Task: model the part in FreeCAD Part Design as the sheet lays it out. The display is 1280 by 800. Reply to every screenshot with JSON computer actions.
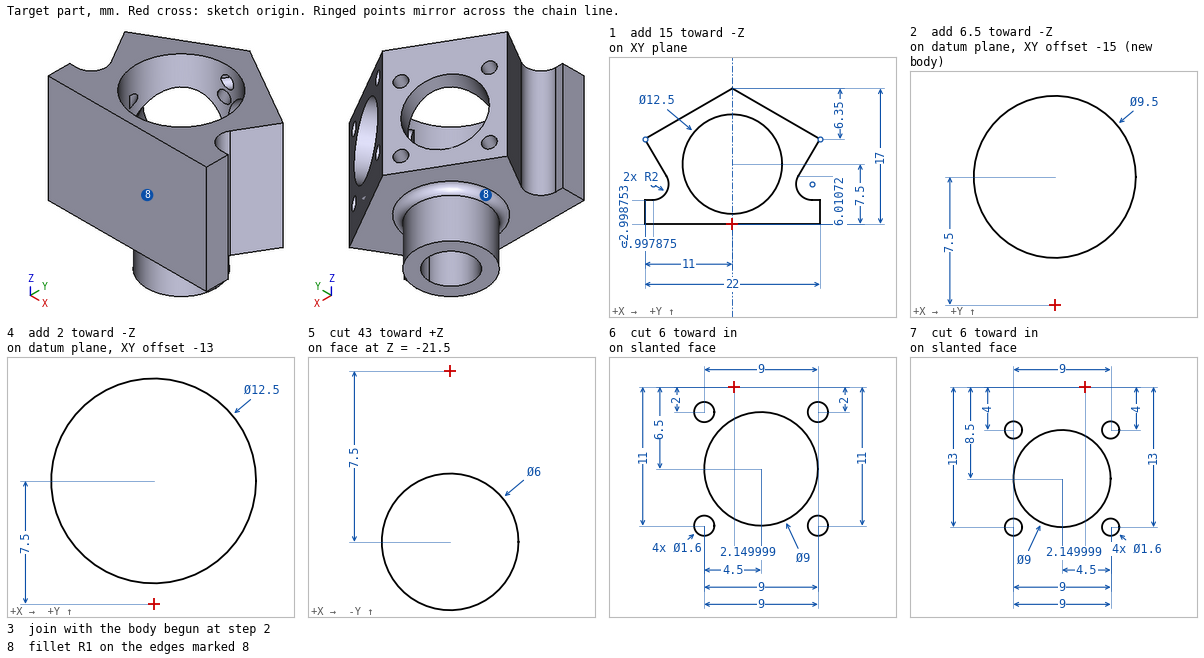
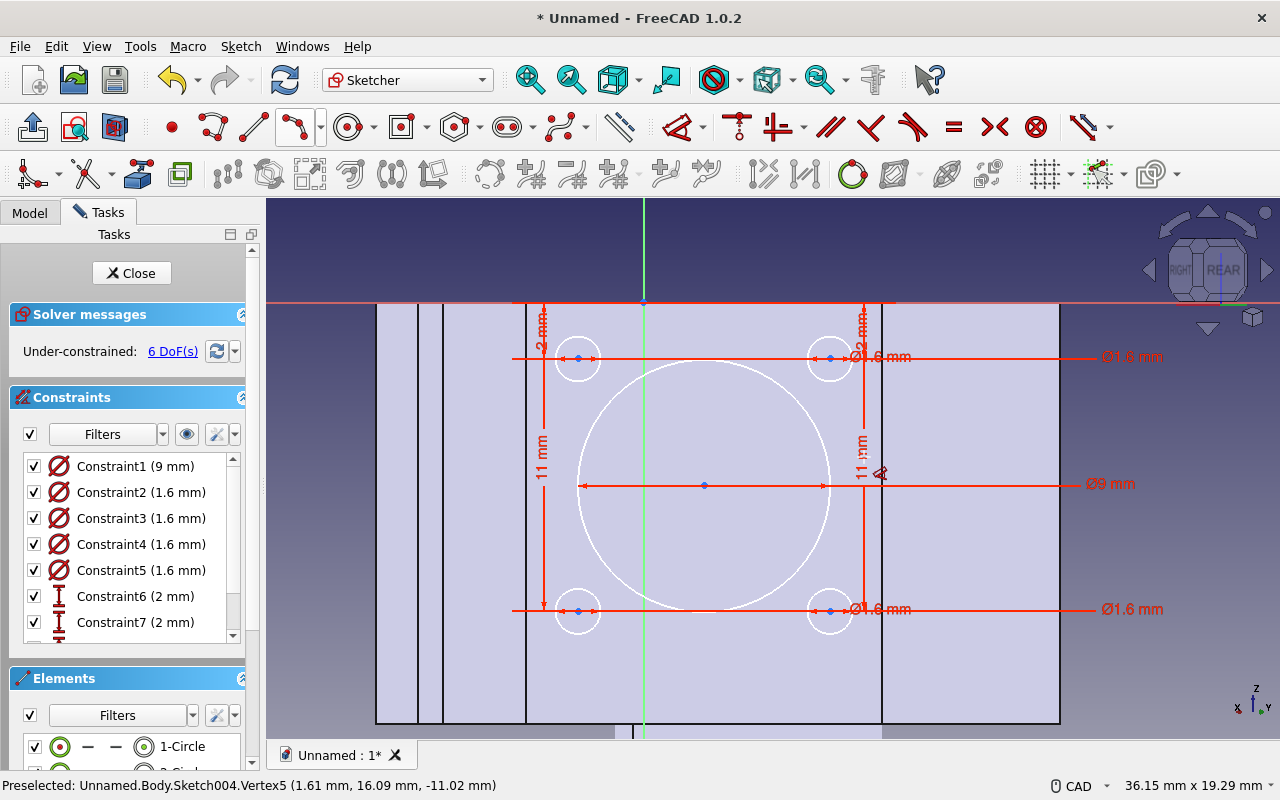
{"action": "left_click", "coordinate": [578, 359]}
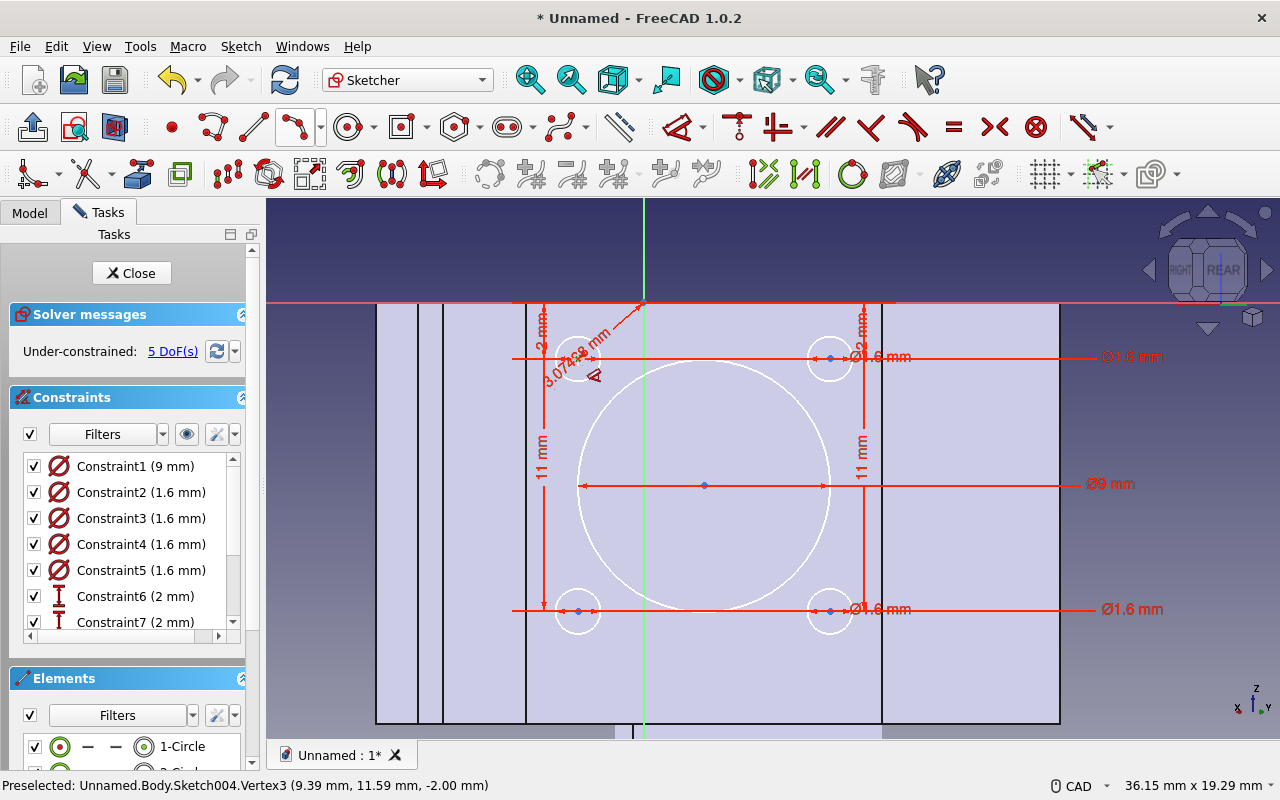
{"action": "left_click", "coordinate": [830, 359]}
{"action": "left_click", "coordinate": [704, 325]}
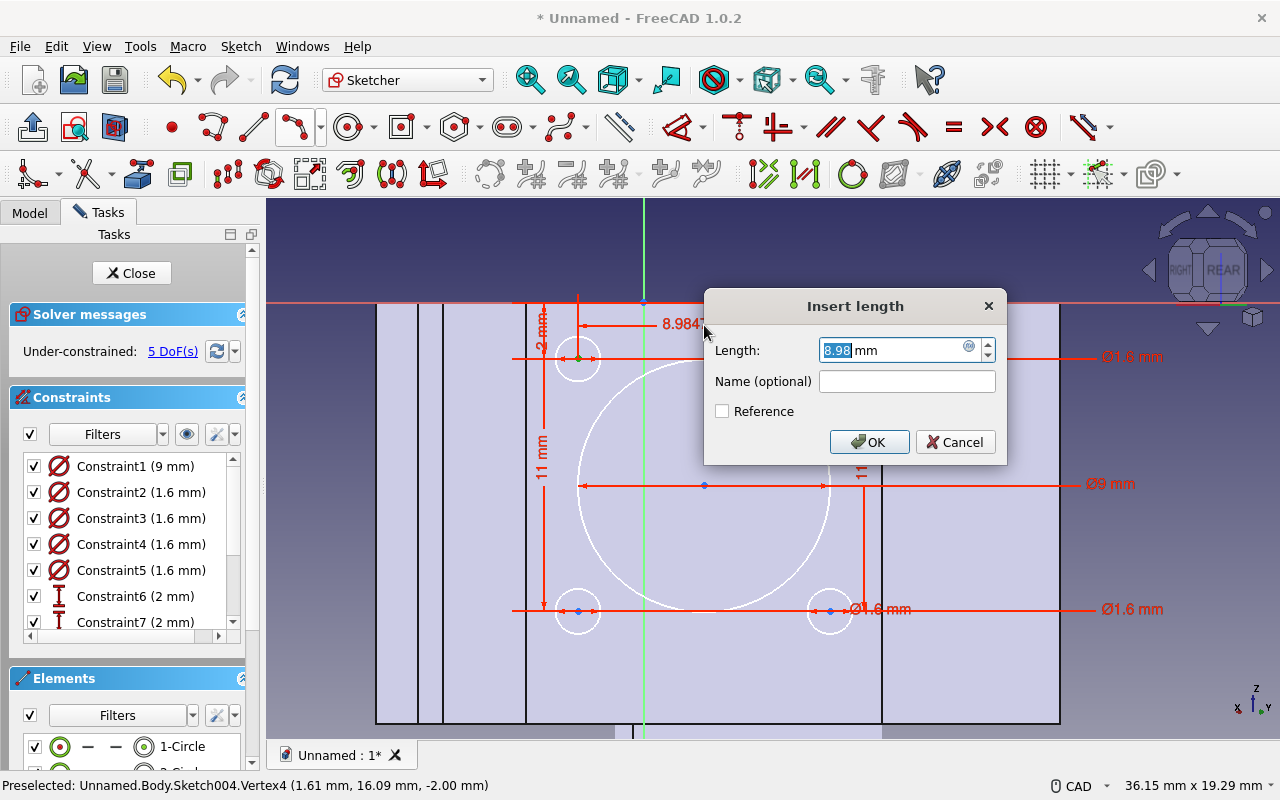
{"action": "type", "text": "9"}
{"action": "key", "text": "Return"}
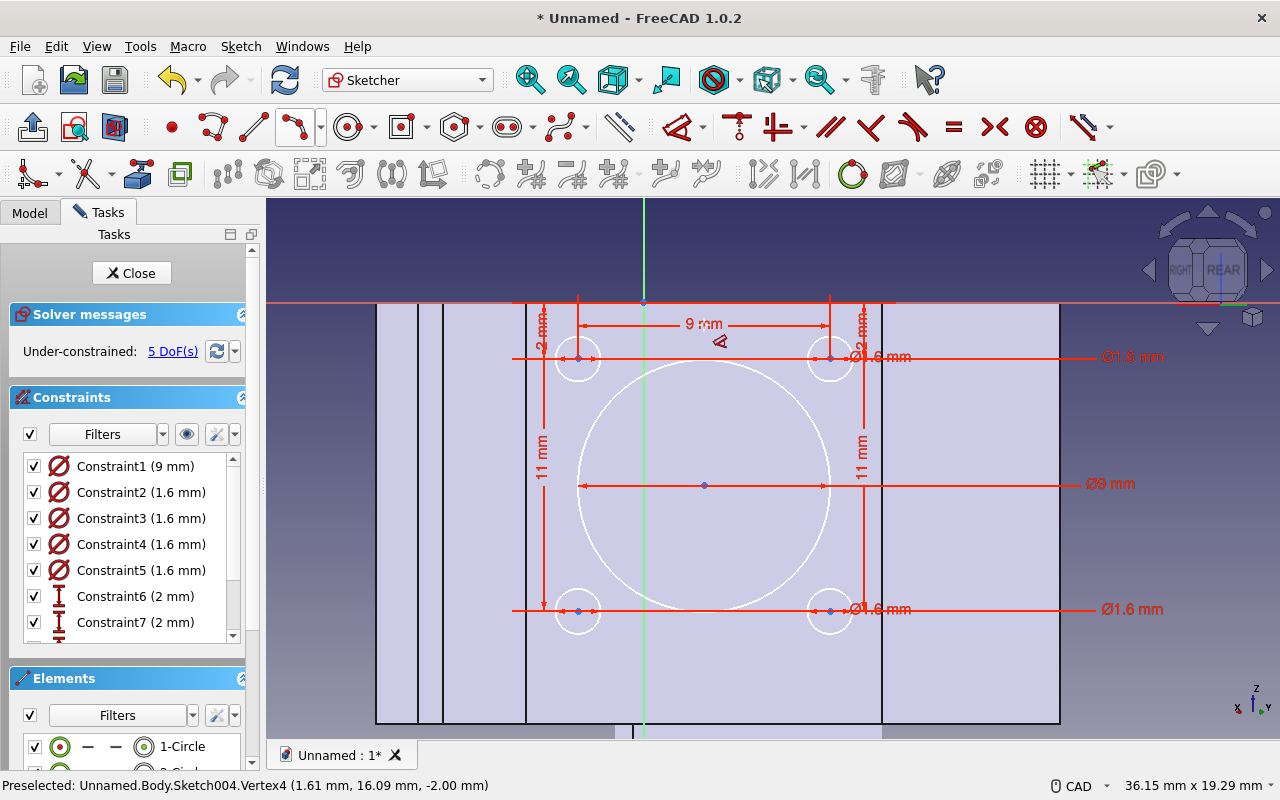
{"action": "left_click", "coordinate": [578, 611]}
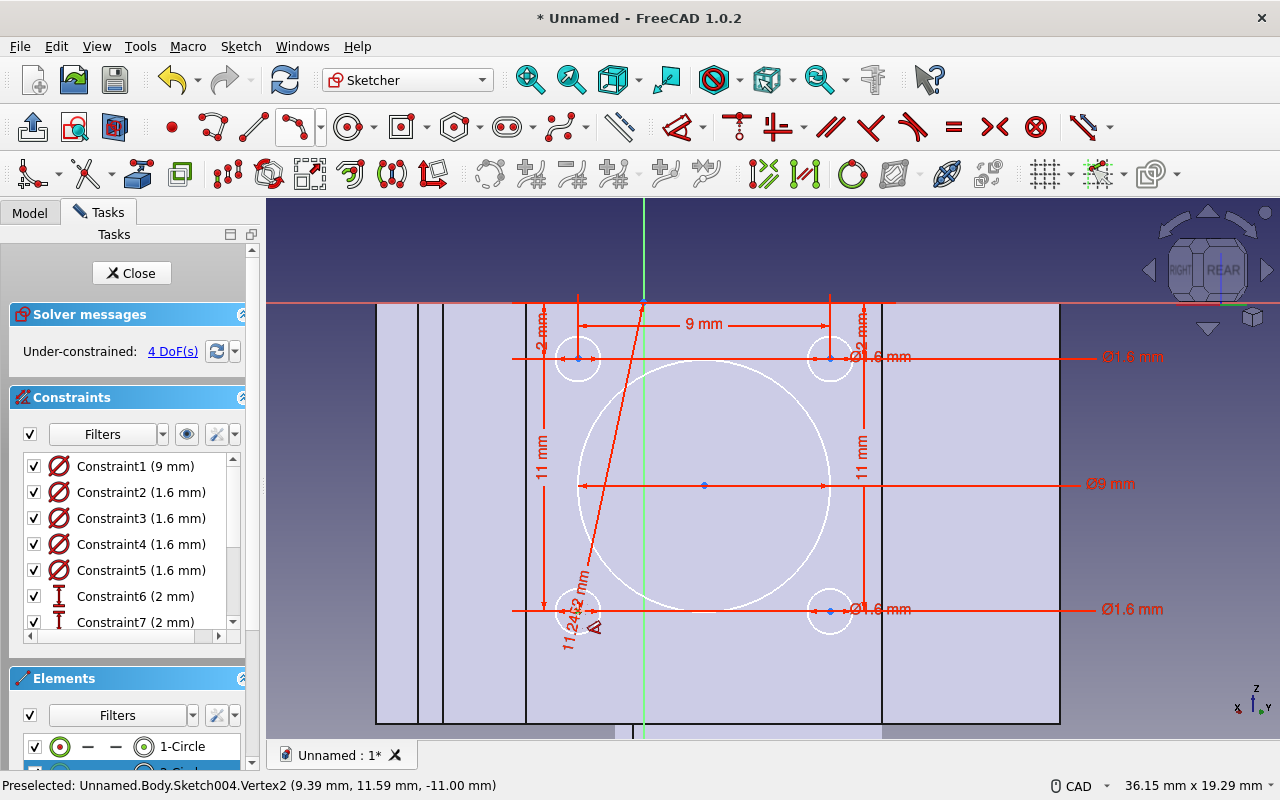
{"action": "left_click", "coordinate": [830, 359]}
{"action": "left_click", "coordinate": [704, 645]}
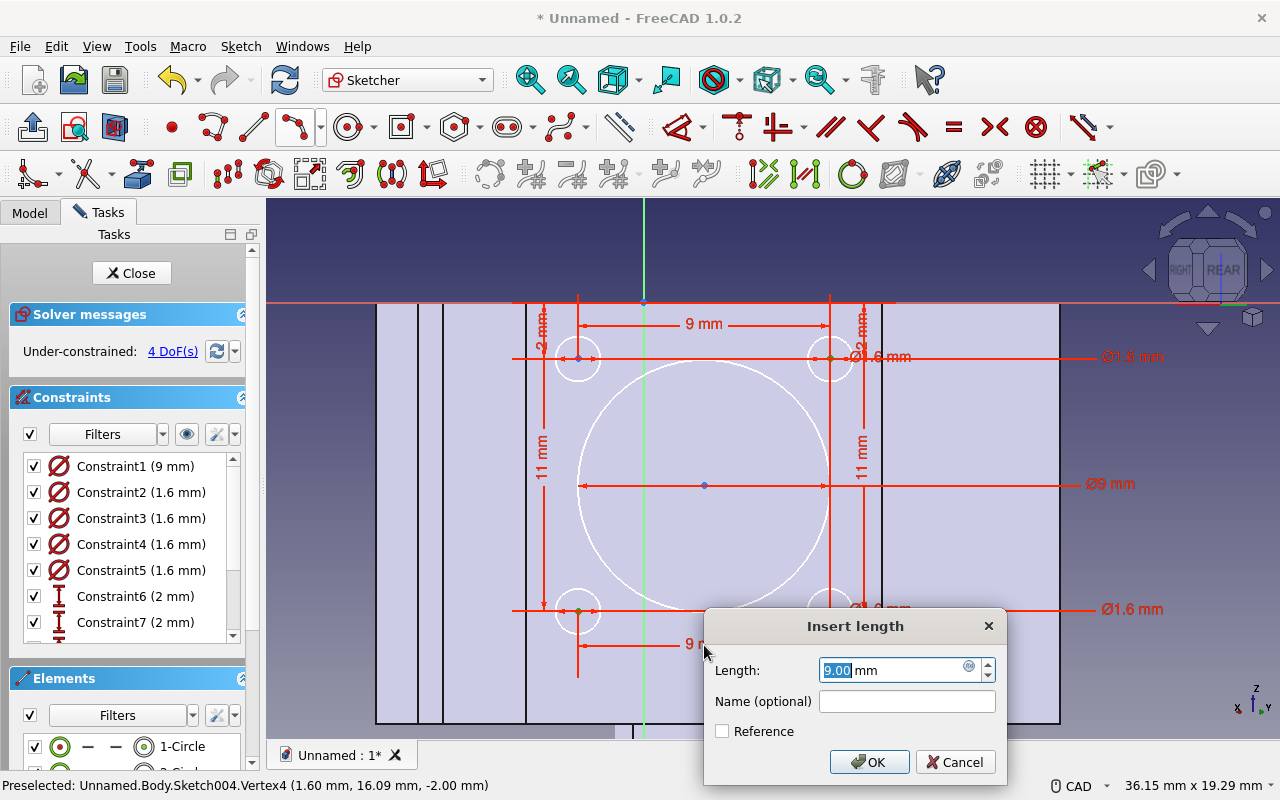
{"action": "type", "text": "9"}
{"action": "key", "text": "Return"}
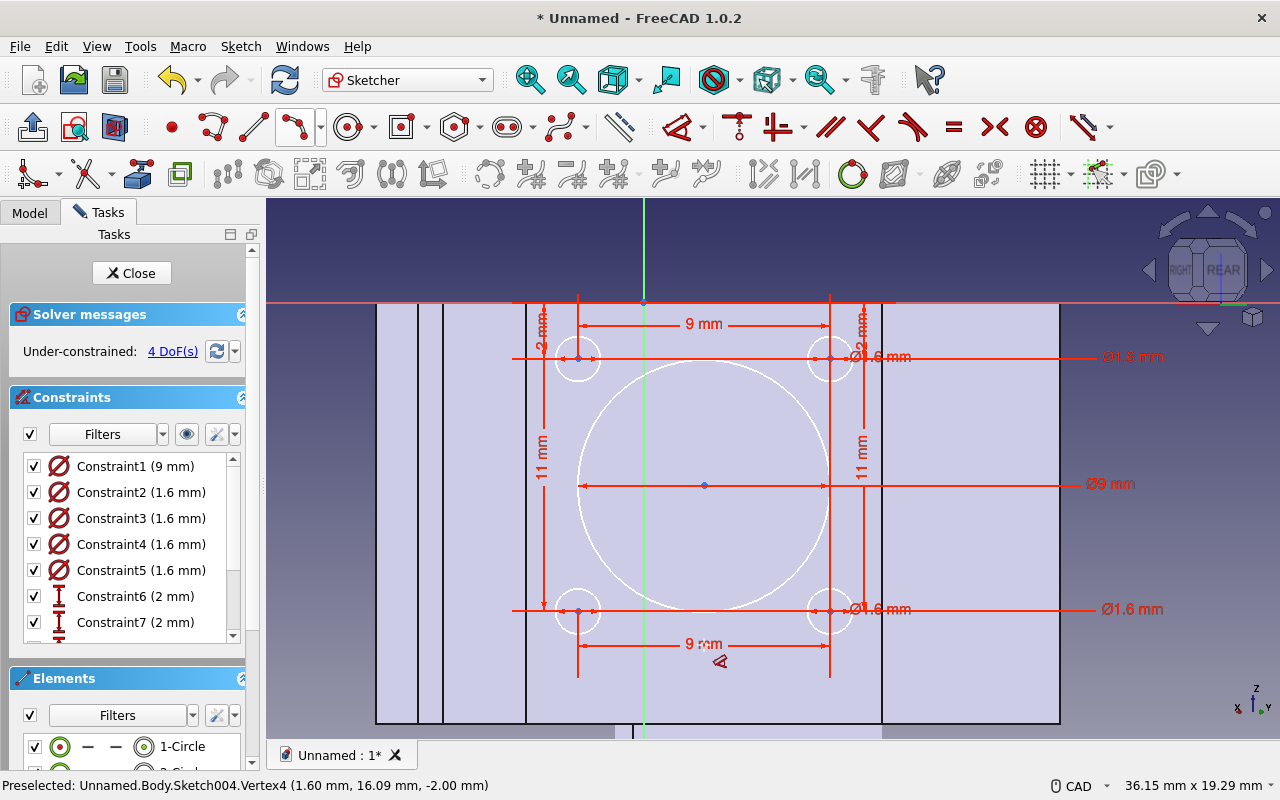
{"action": "left_click", "coordinate": [578, 611]}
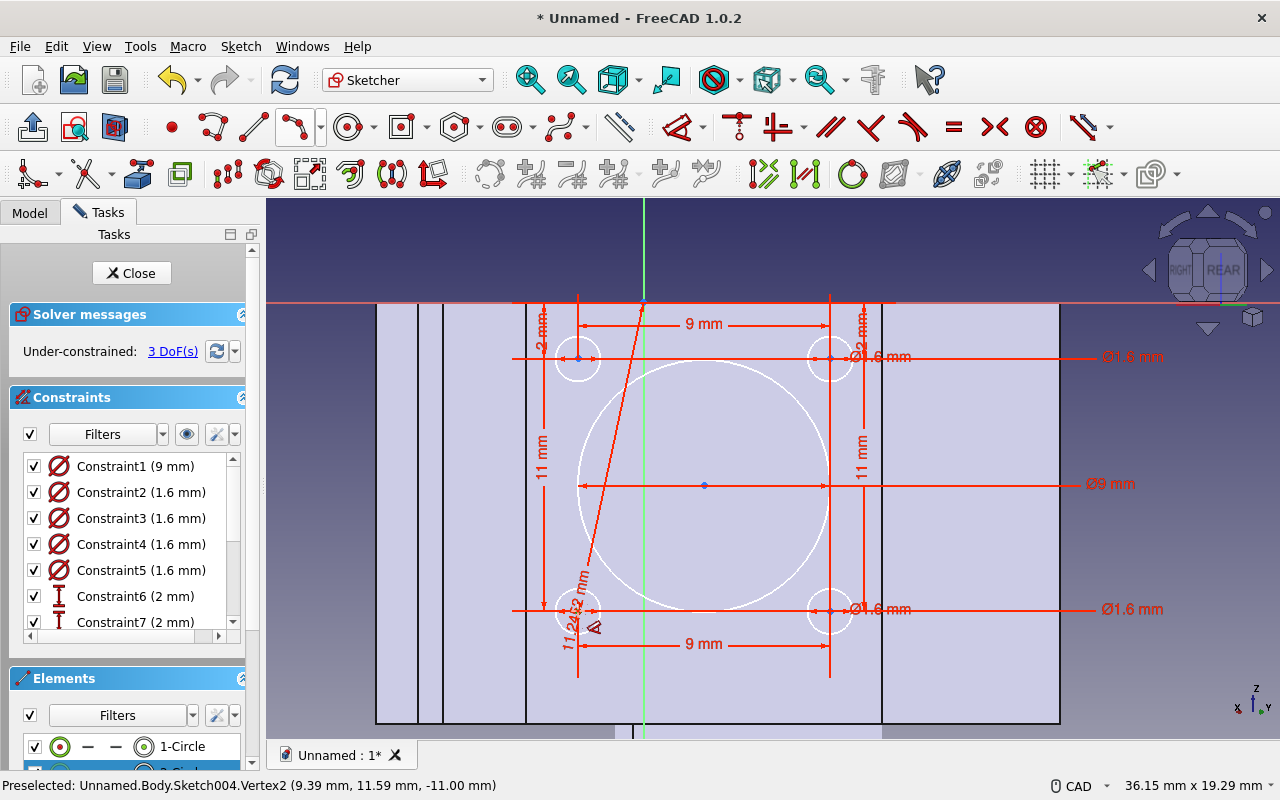
{"action": "left_click", "coordinate": [830, 611]}
{"action": "left_click", "coordinate": [616, 645]}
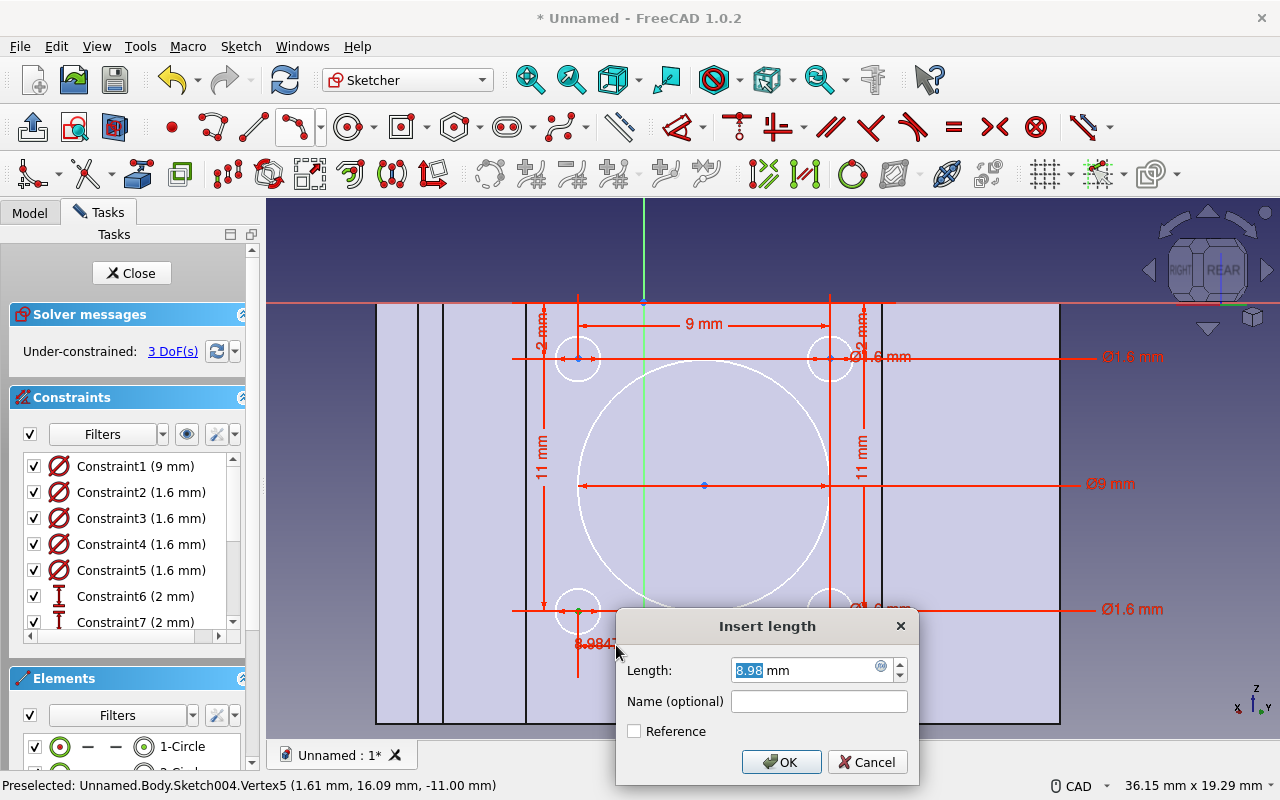
{"action": "type", "text": "9"}
{"action": "key", "text": "Return"}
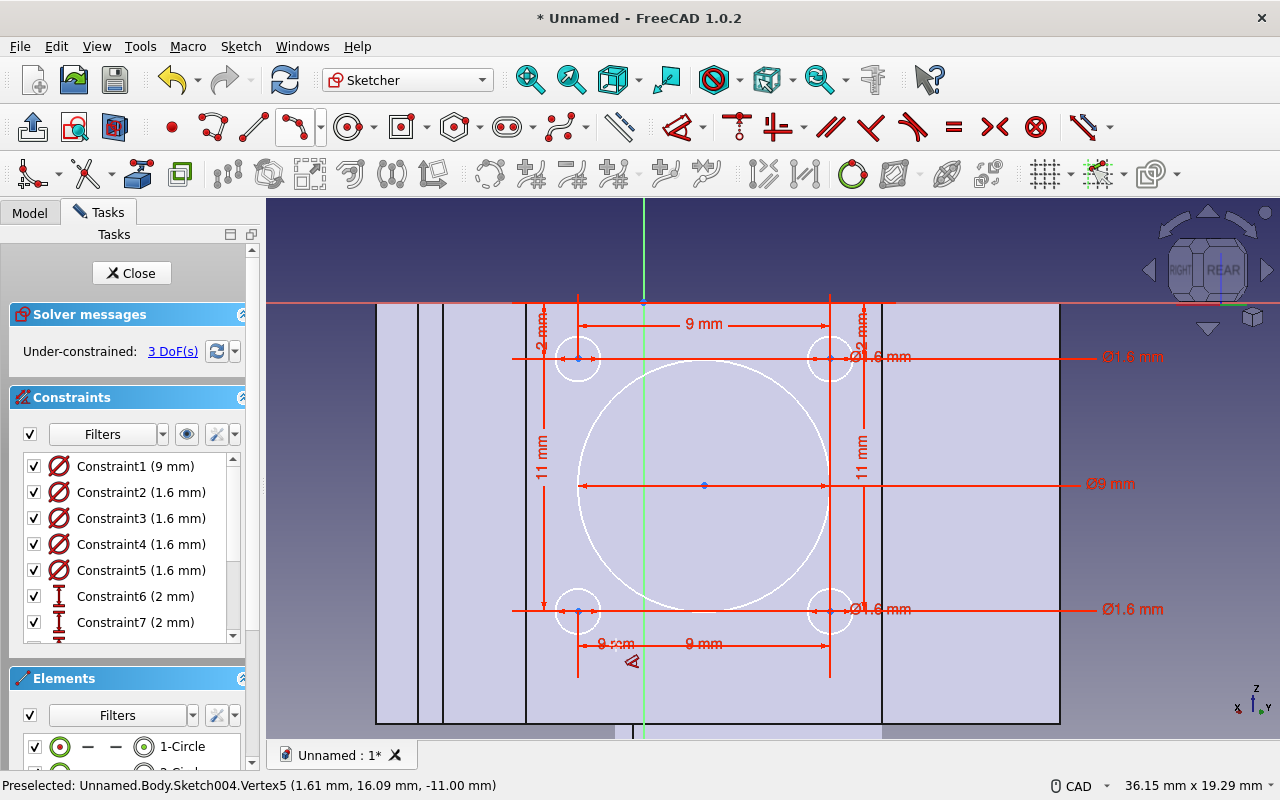
{"action": "left_click", "coordinate": [704, 486]}
{"action": "left_click", "coordinate": [610, 437]}